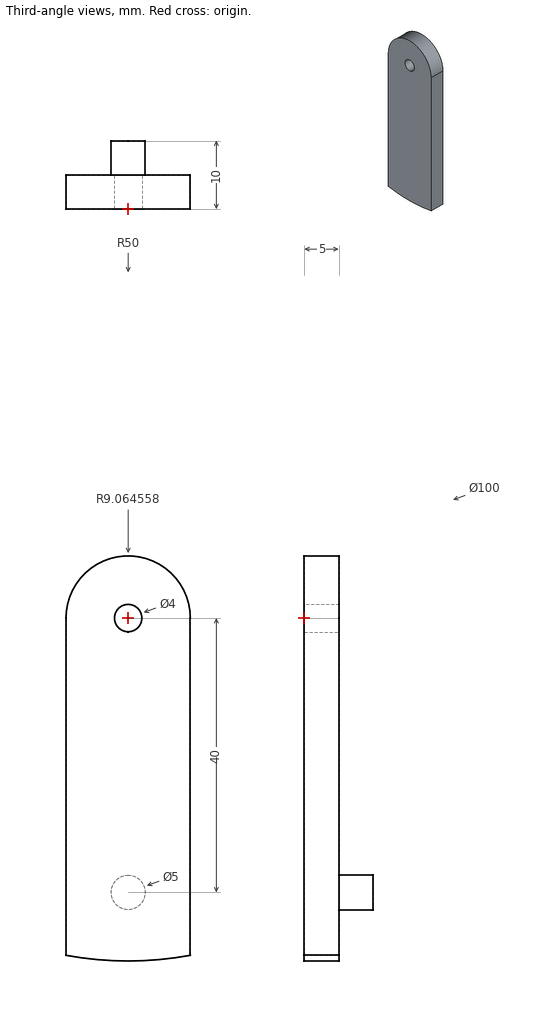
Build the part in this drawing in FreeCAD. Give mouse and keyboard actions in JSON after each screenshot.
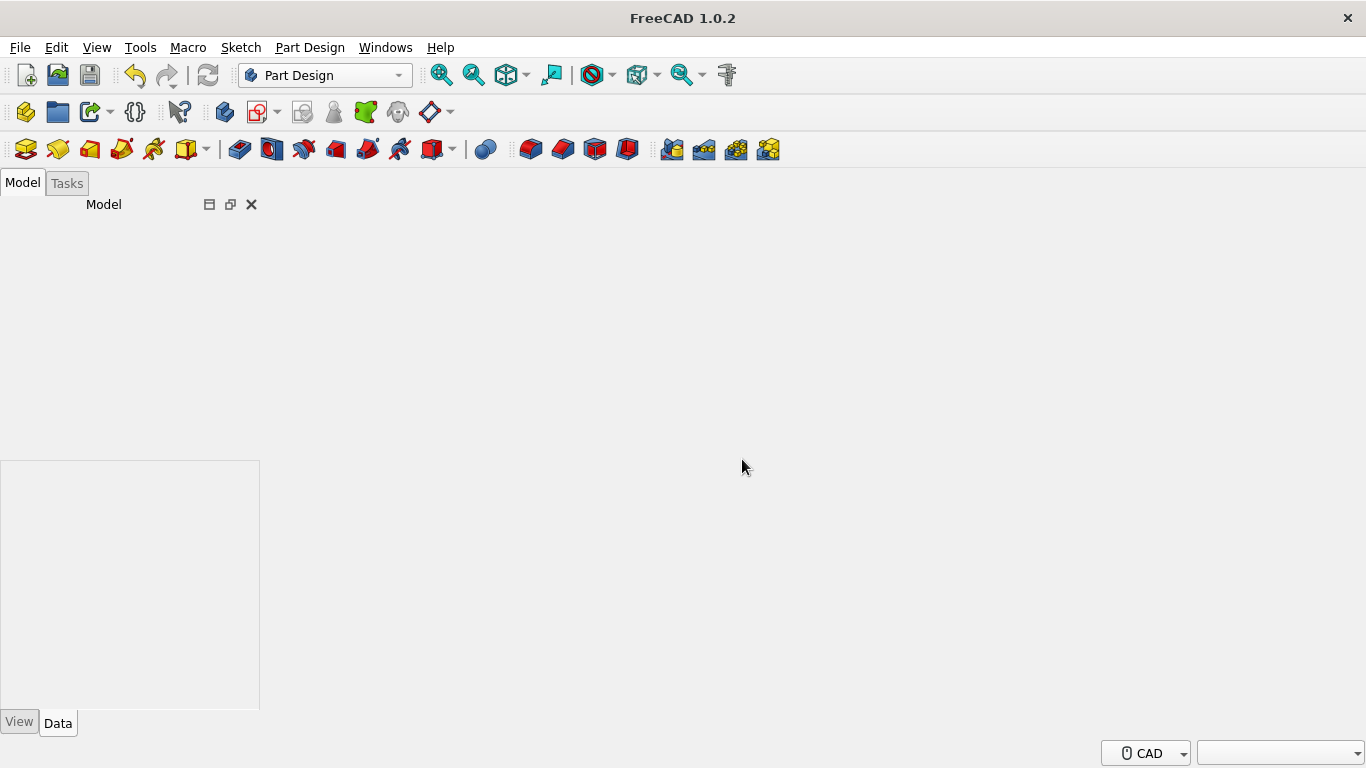
{"action": "left_click", "coordinate": [26, 76]}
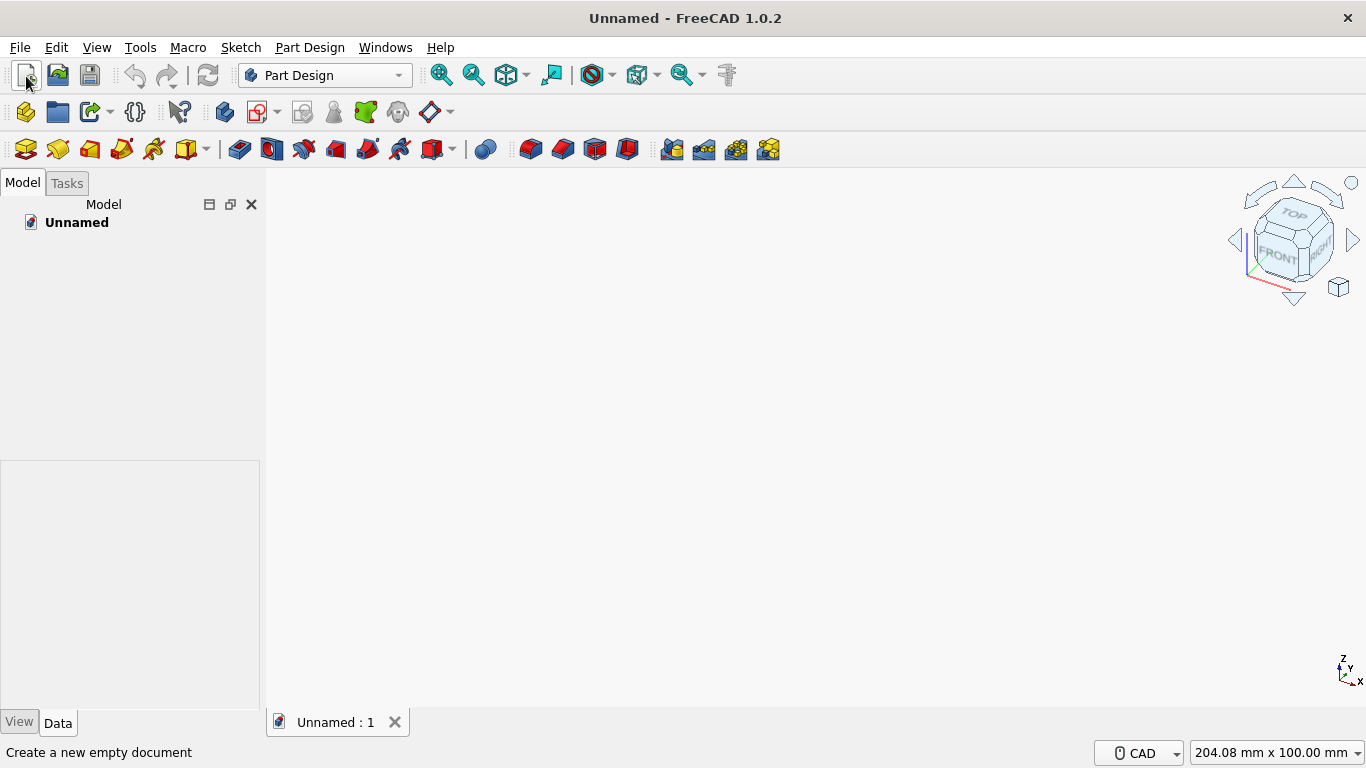
{"action": "left_click", "coordinate": [258, 112]}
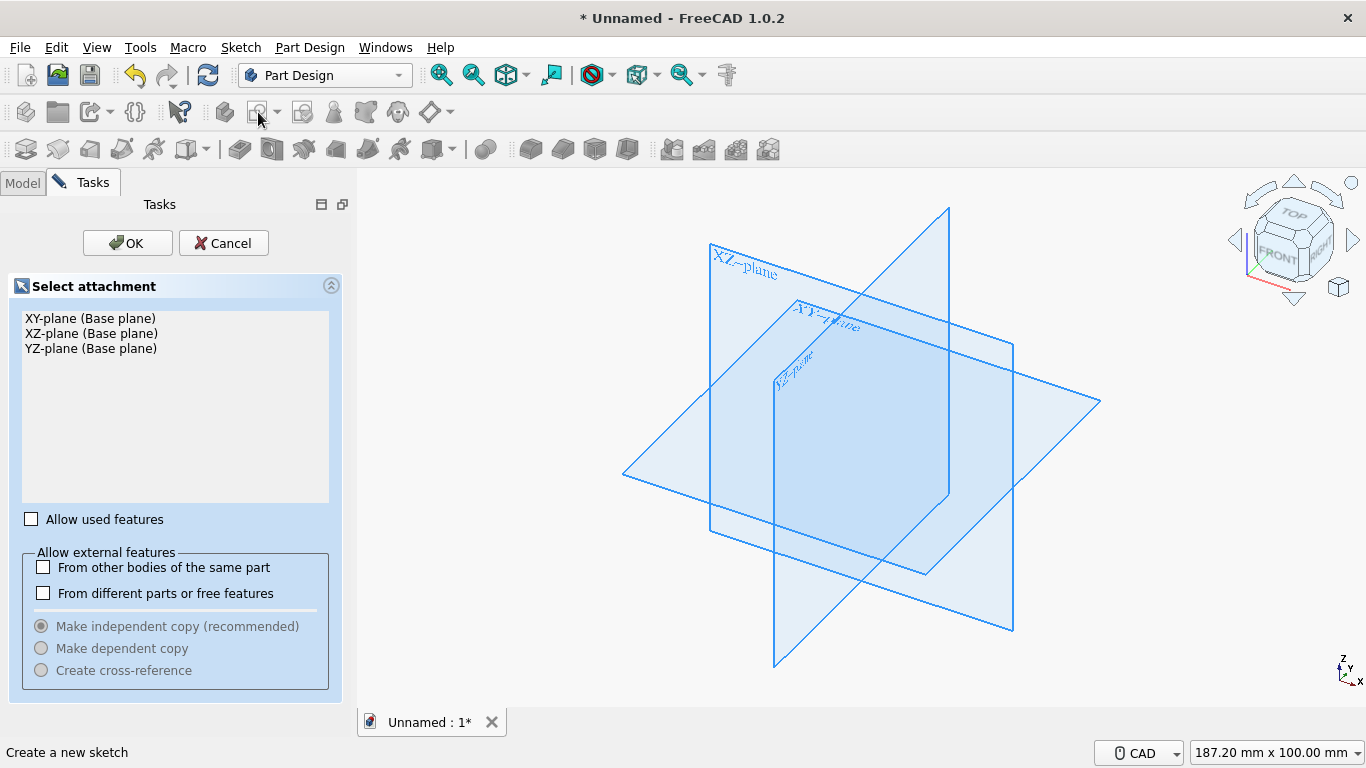
{"action": "left_click", "coordinate": [82, 334]}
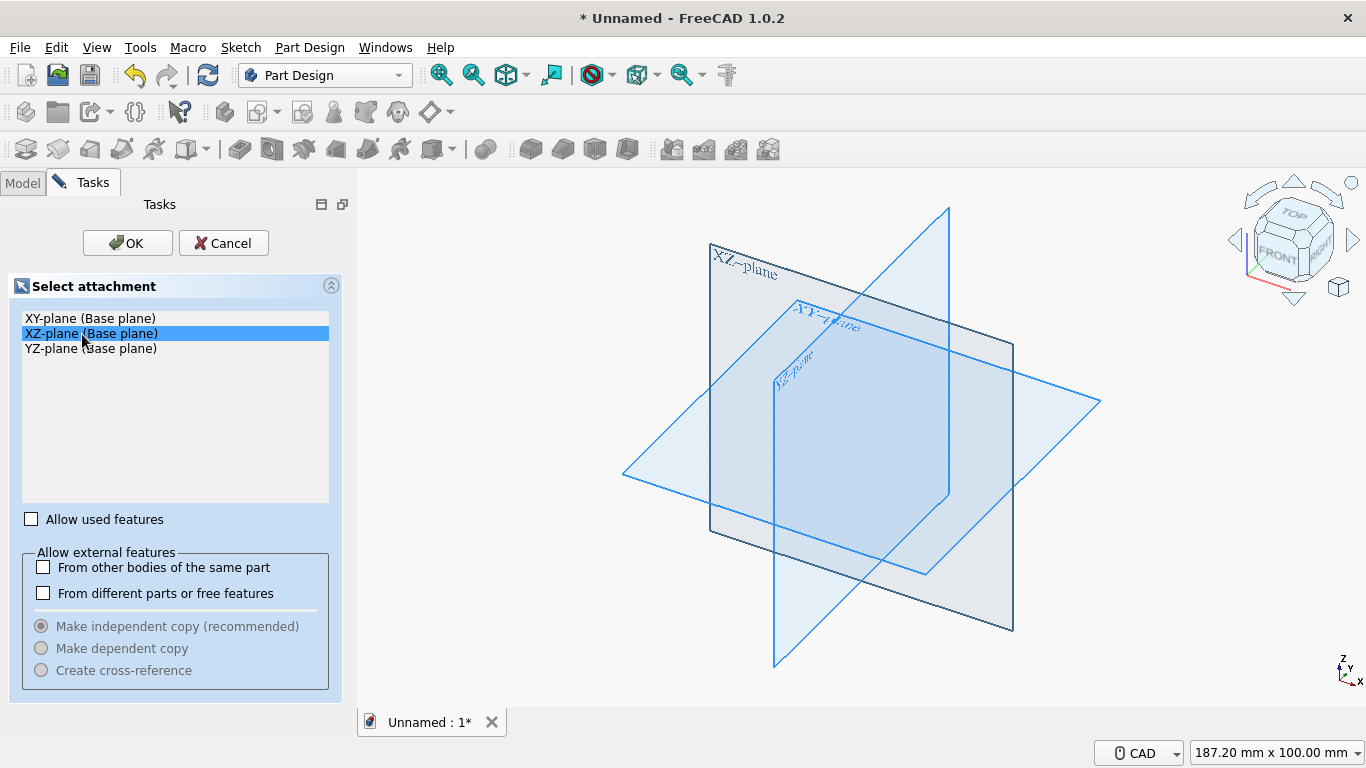
{"action": "left_click", "coordinate": [128, 243]}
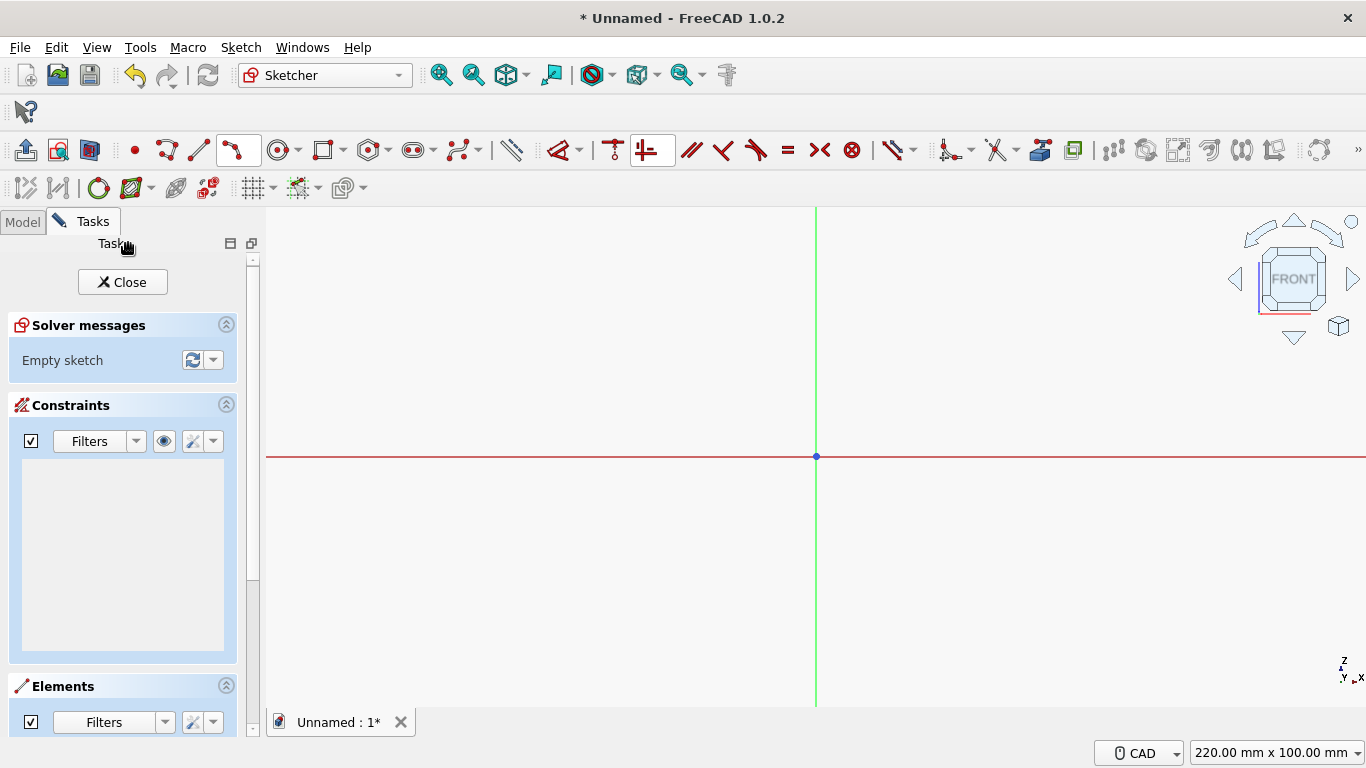
{"action": "scroll", "coordinate": [608, 457], "scroll_direction": "down", "scroll_amount": 2}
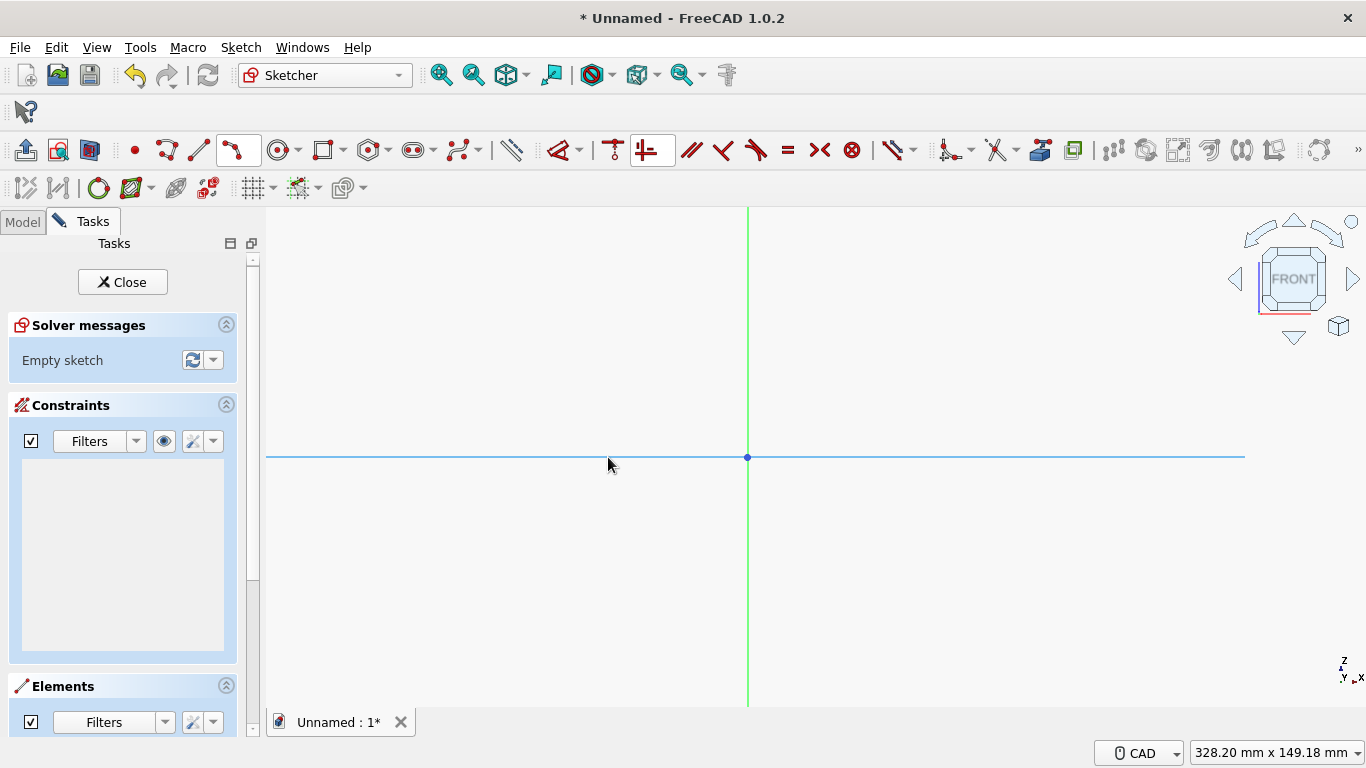
{"action": "left_click", "coordinate": [278, 150]}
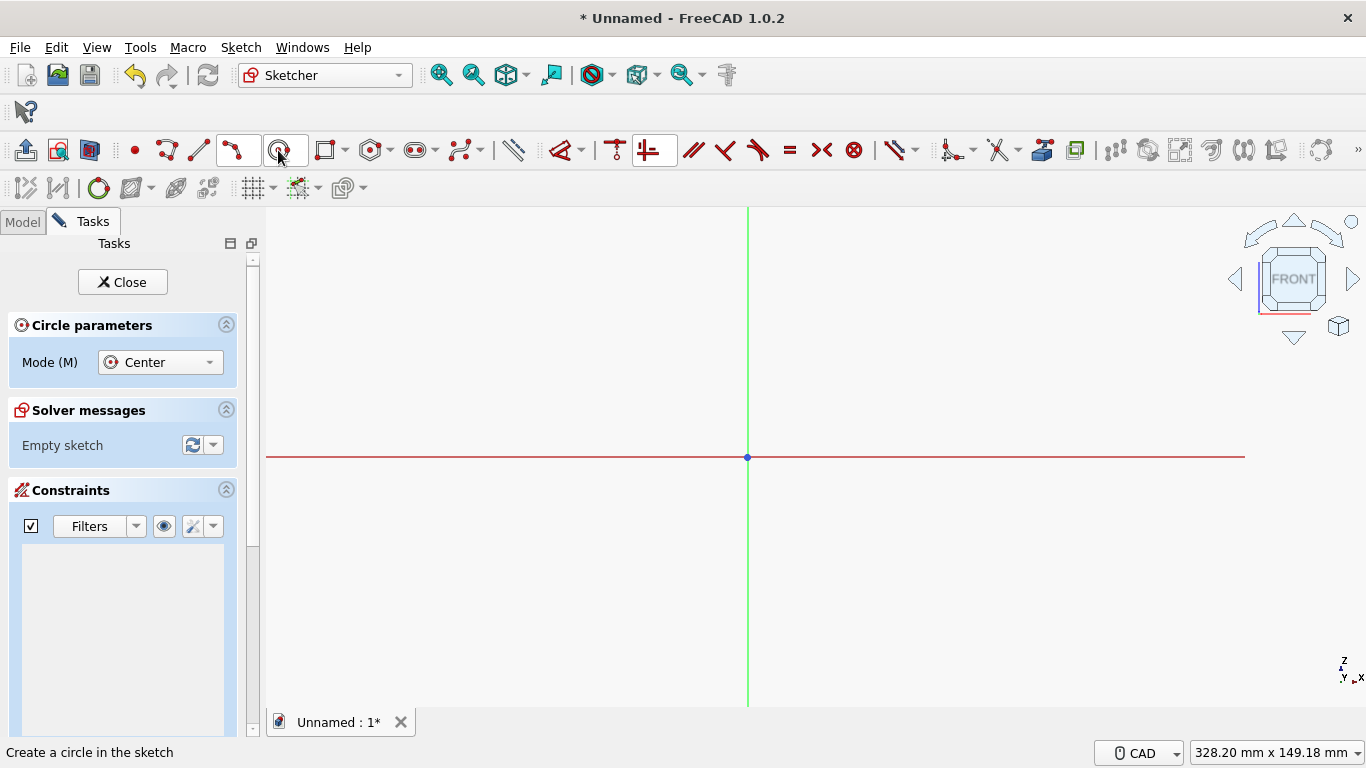
{"action": "left_click", "coordinate": [748, 457]}
{"action": "left_click", "coordinate": [866, 339]}
{"action": "key", "text": "Escape"}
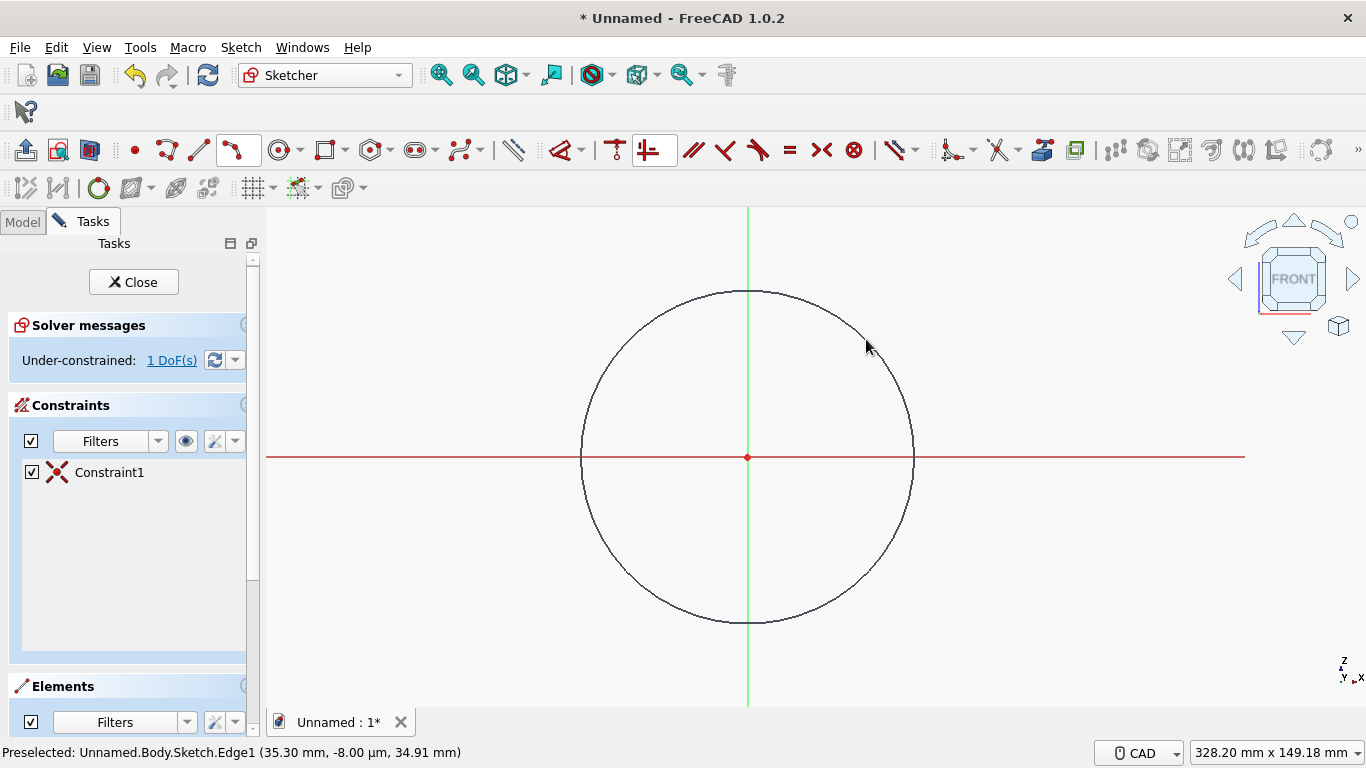
{"action": "left_click", "coordinate": [865, 339]}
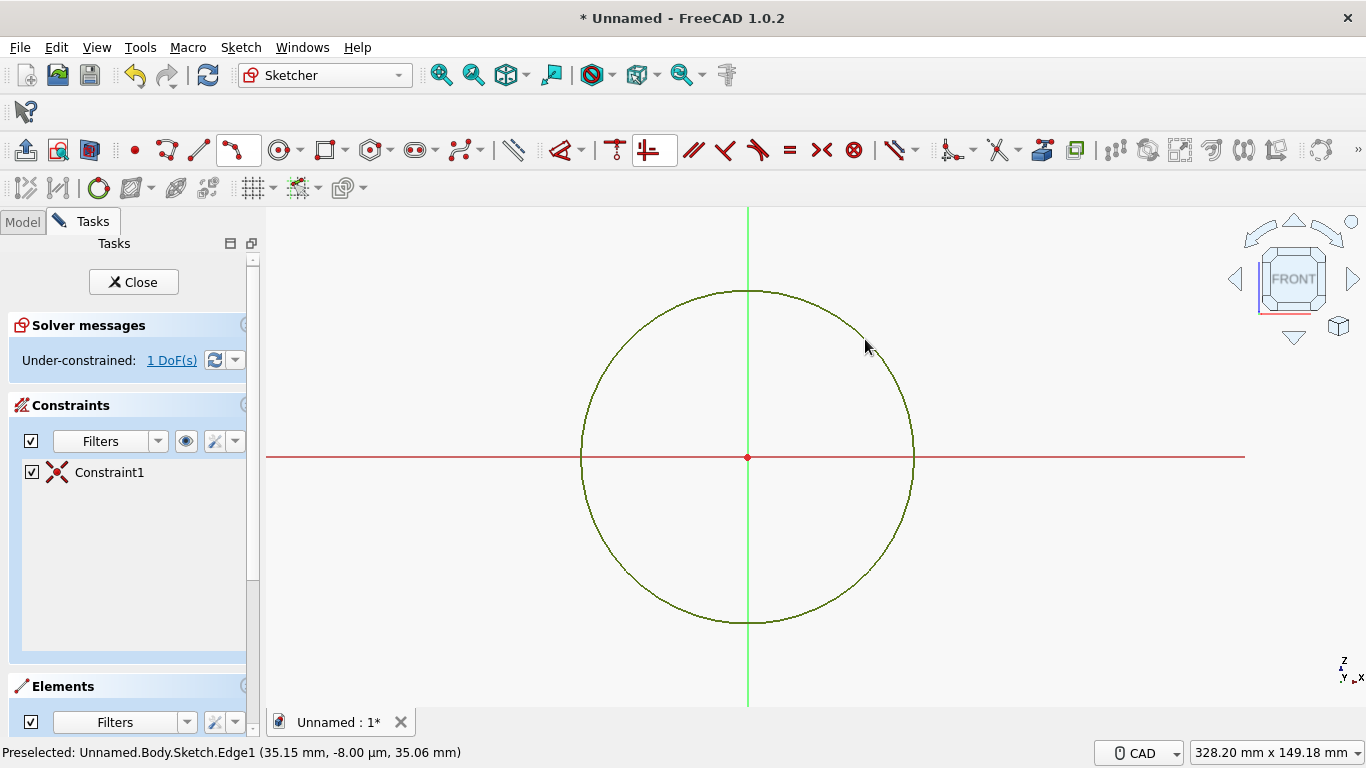
{"action": "key", "text": "k o"}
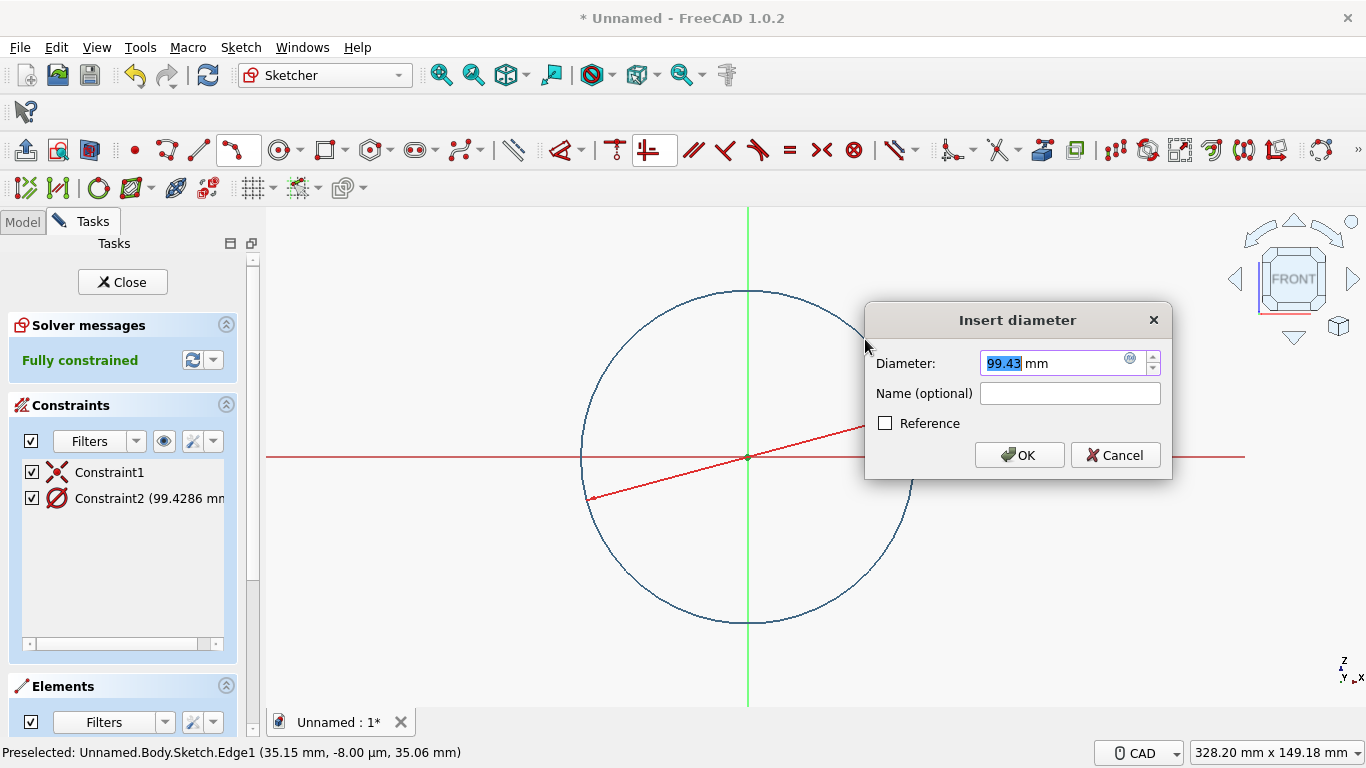
{"action": "type", "text": "100"}
{"action": "key", "text": "Return"}